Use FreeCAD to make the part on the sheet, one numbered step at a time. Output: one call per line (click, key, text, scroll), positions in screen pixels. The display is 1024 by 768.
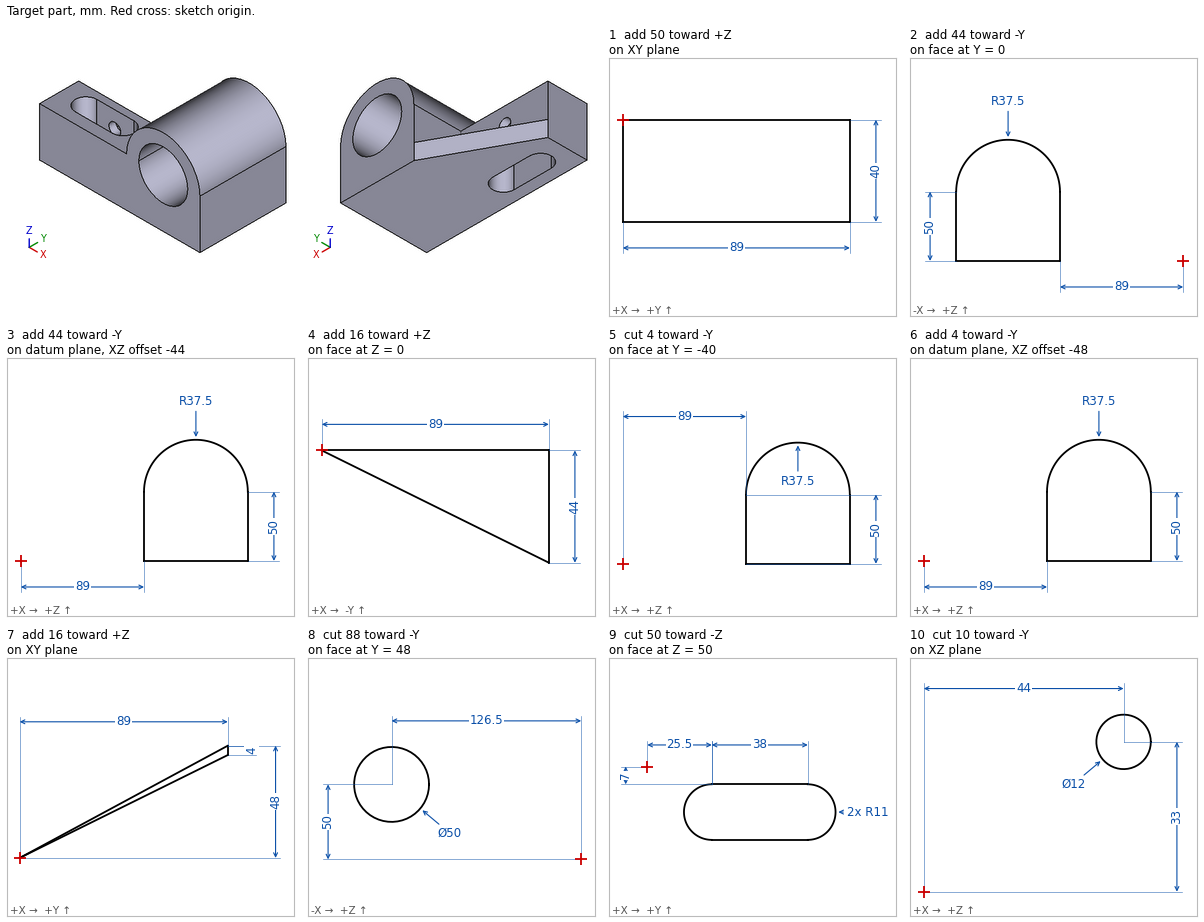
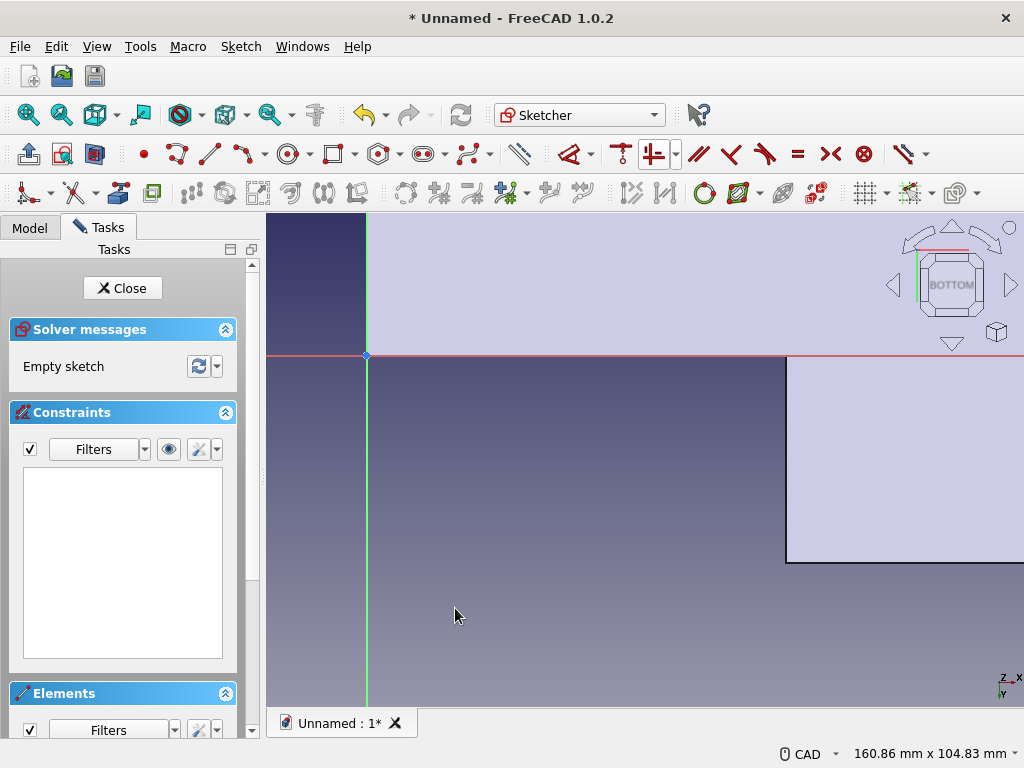
key(g)
key(m)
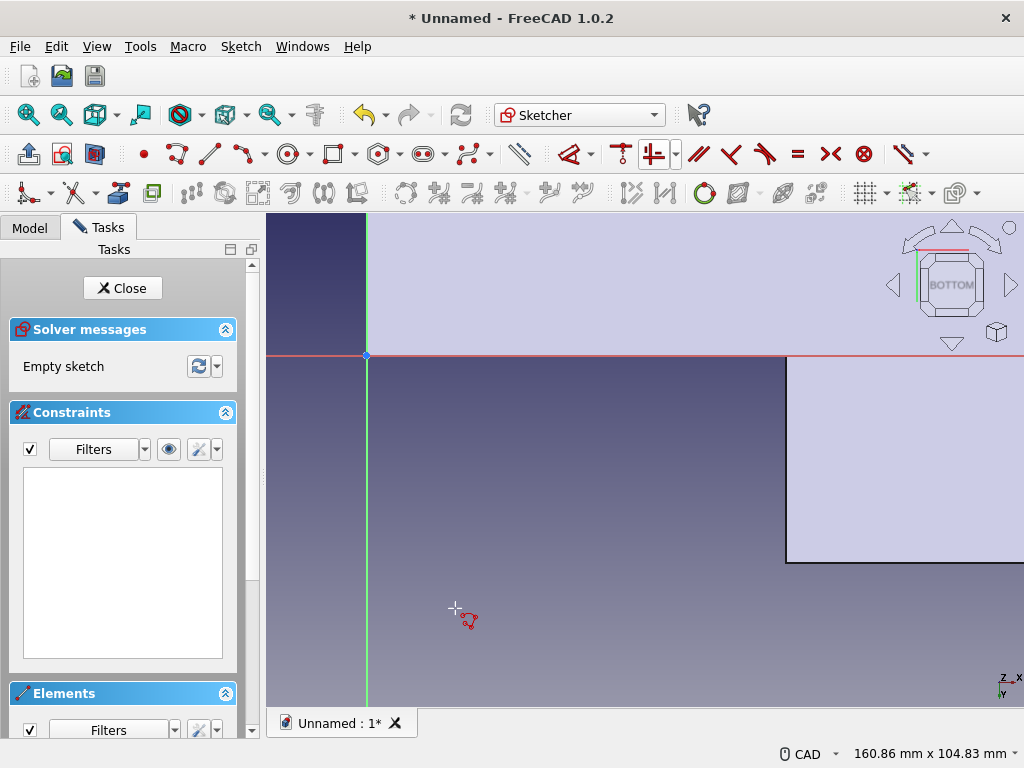
click(367, 356)
click(786, 563)
click(786, 365)
click(367, 356)
key(Escape)
key(Escape)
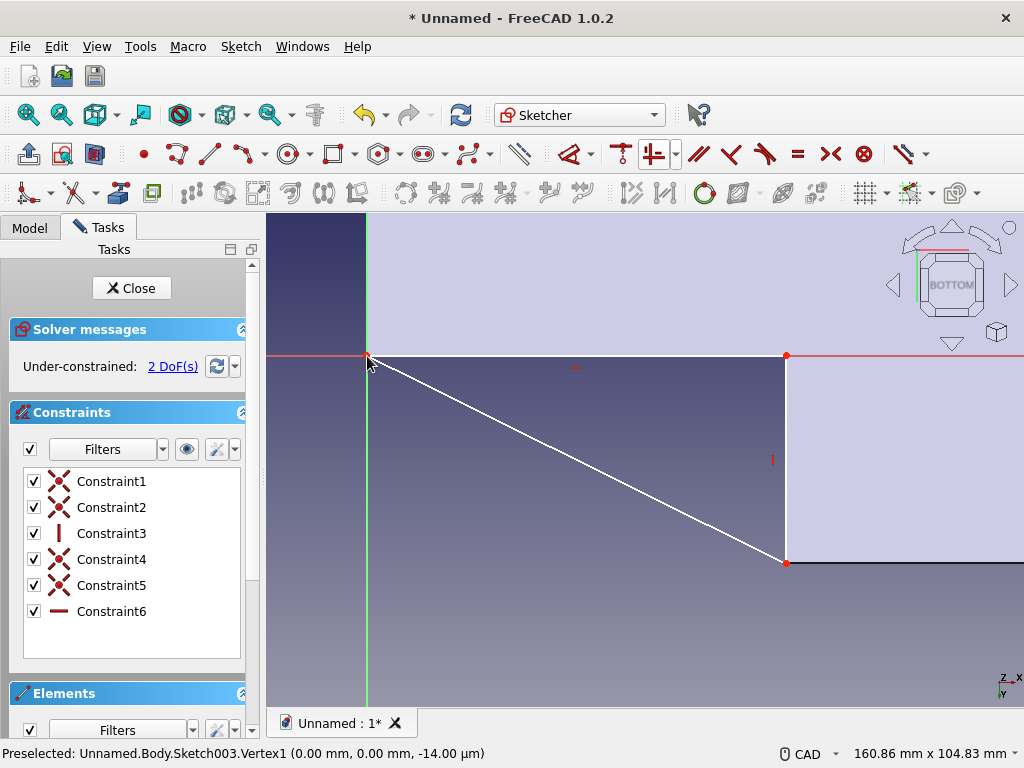
click(568, 154)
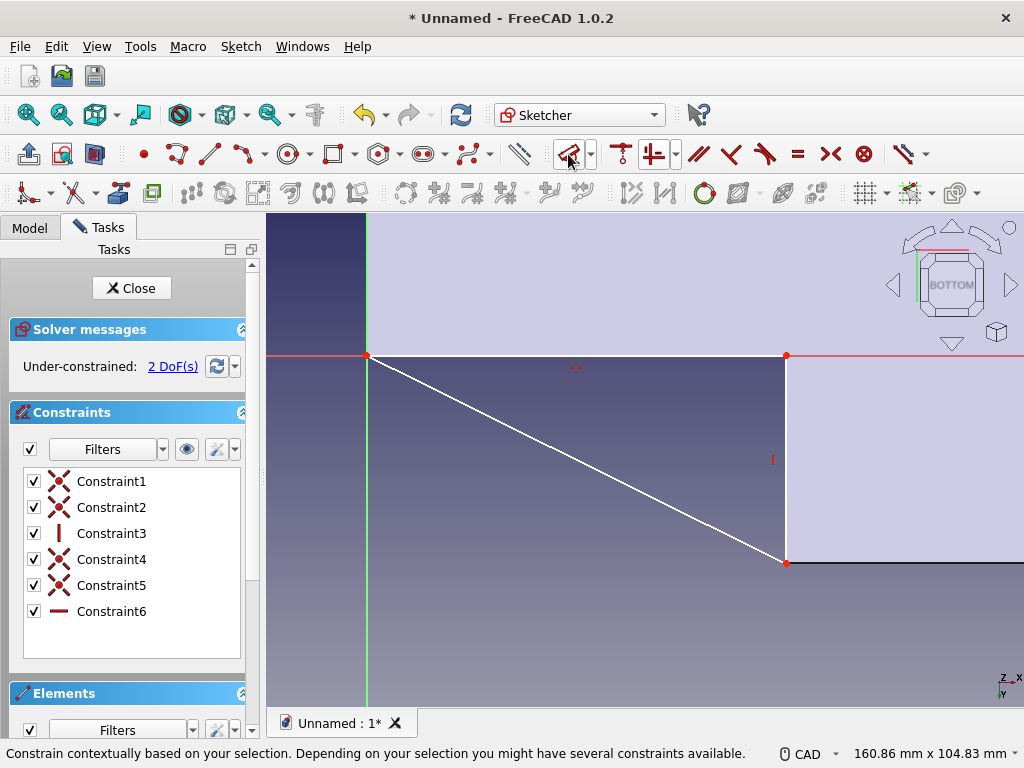
click(786, 501)
click(820, 460)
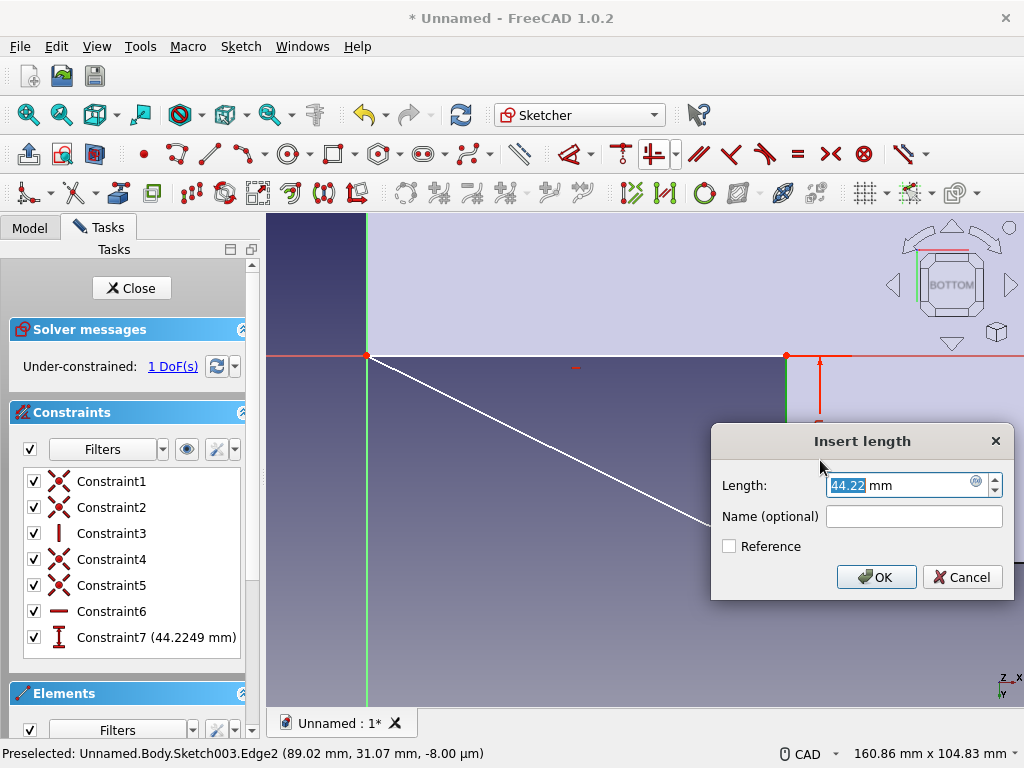
text(44)
key(Return)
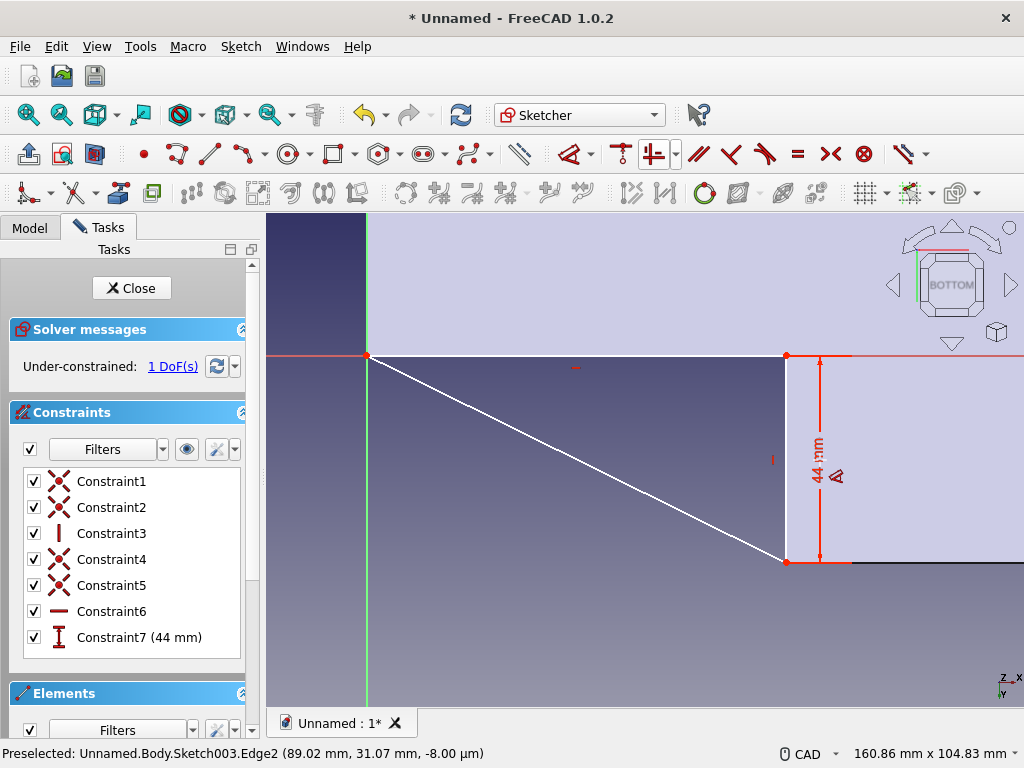
click(660, 356)
click(576, 322)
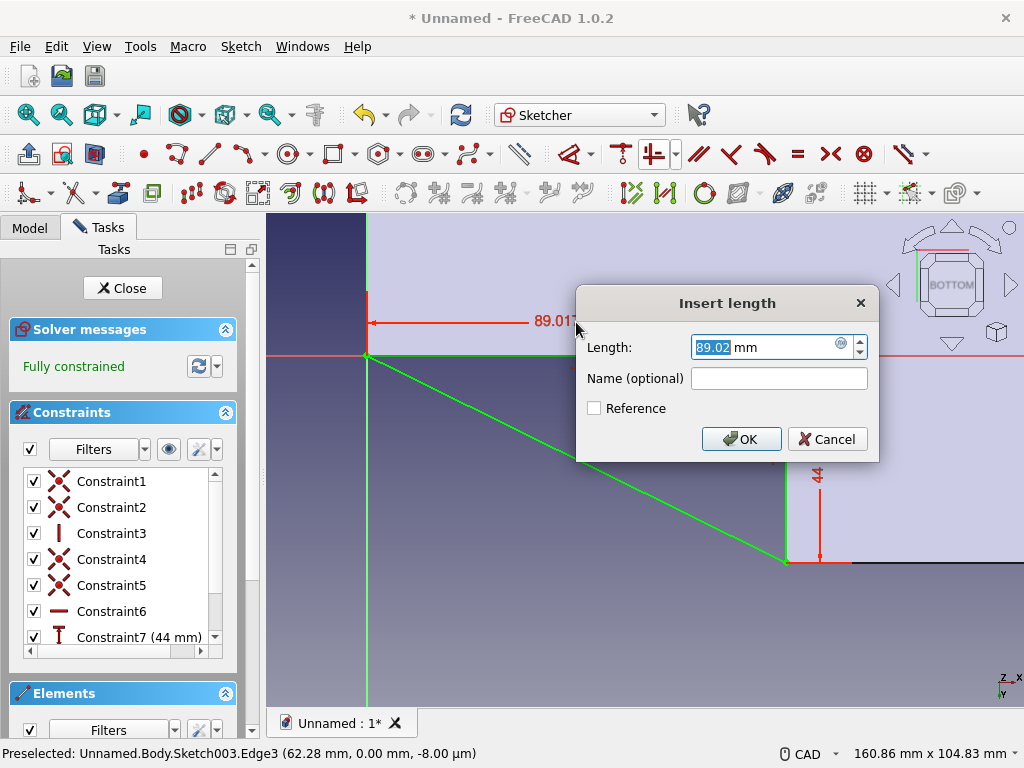
text(89)
key(Return)
key(Escape)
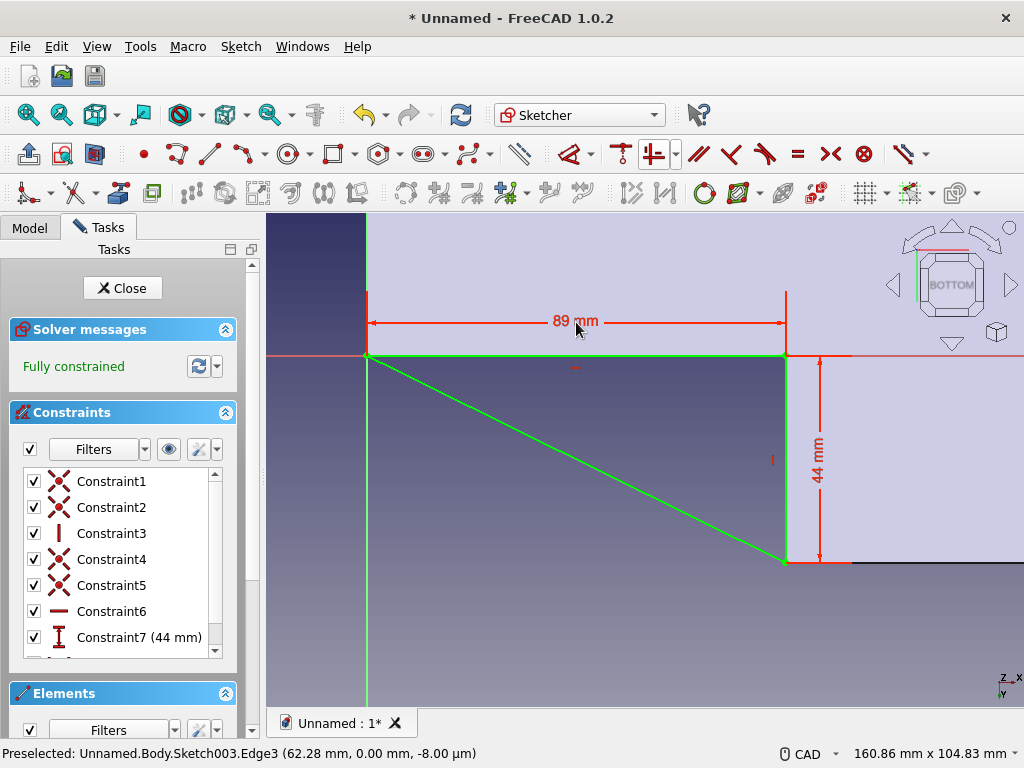
click(123, 288)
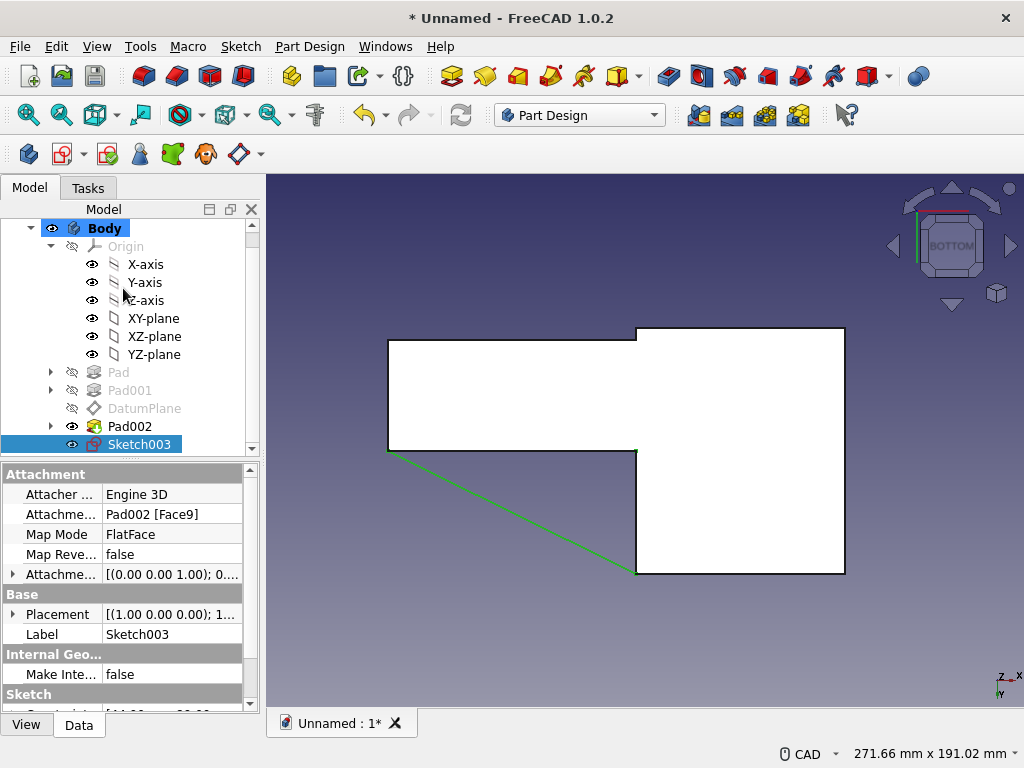
click(452, 76)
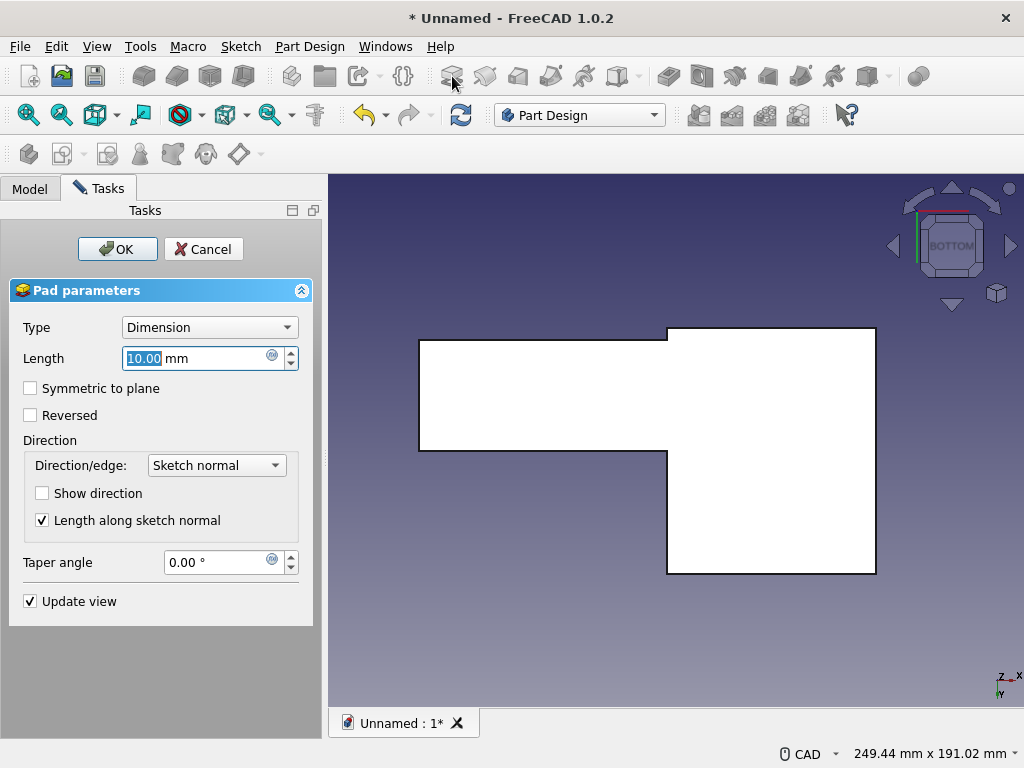
text(16)
key(Tab)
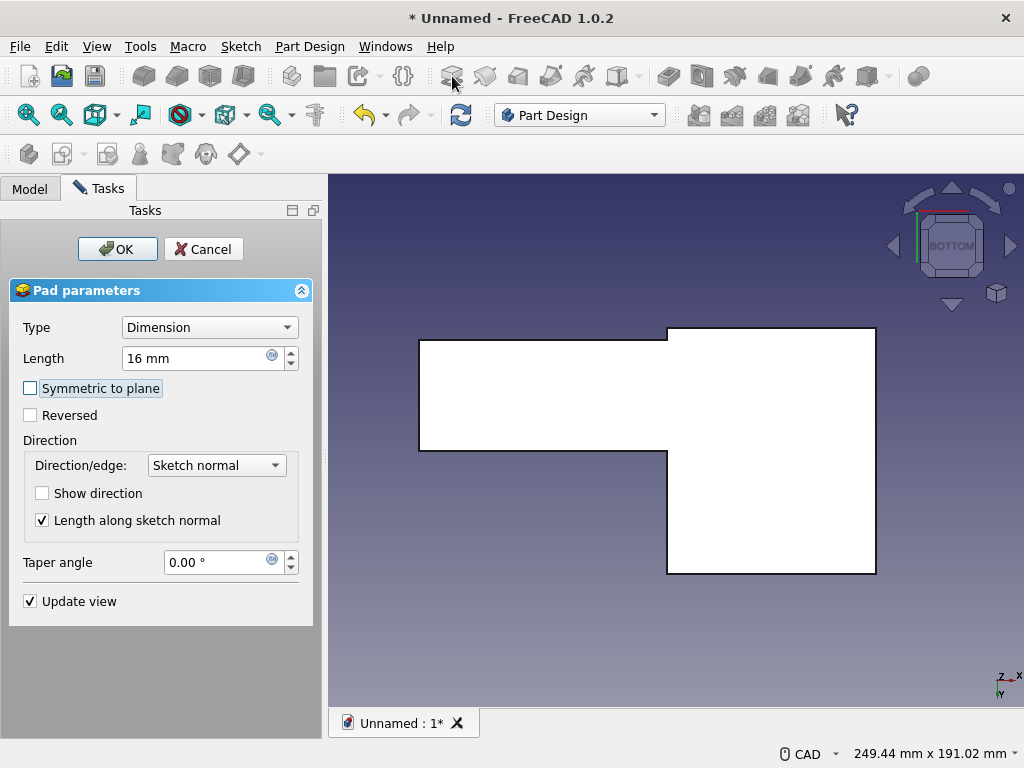
click(31, 415)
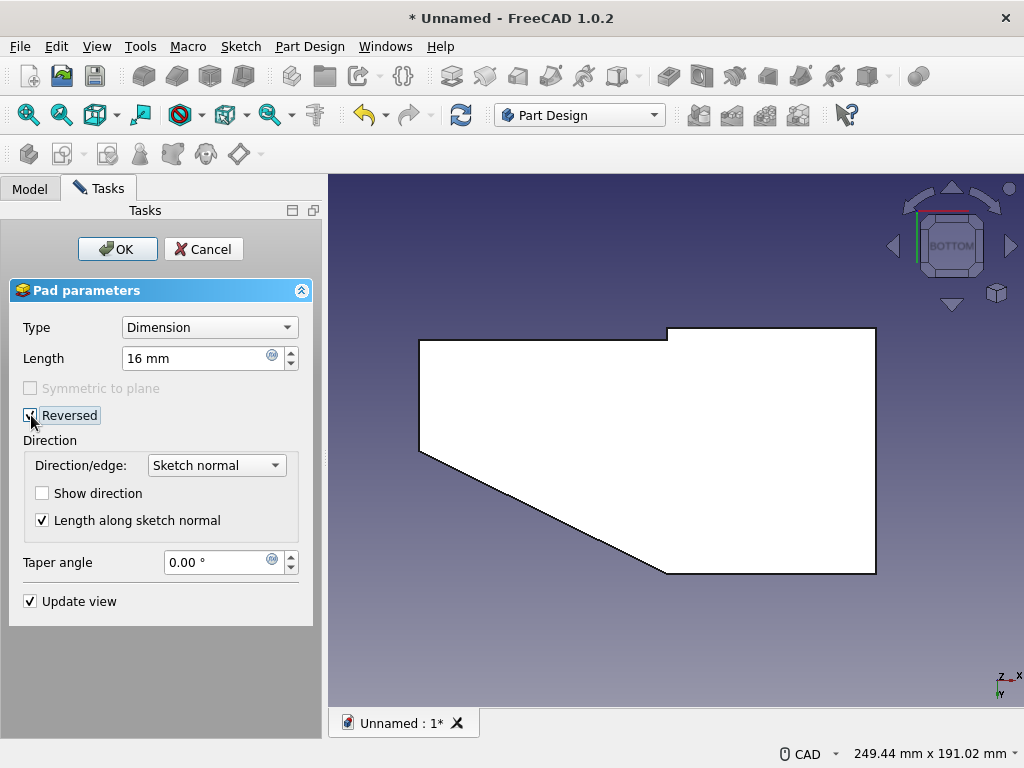
click(118, 249)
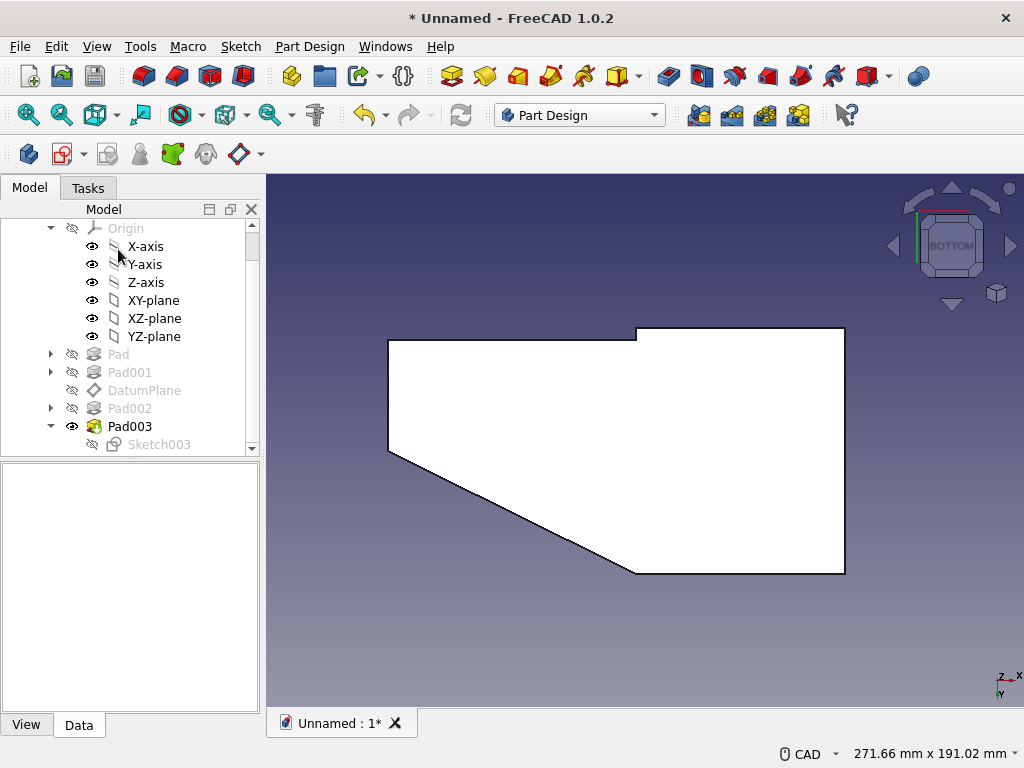
key(0)